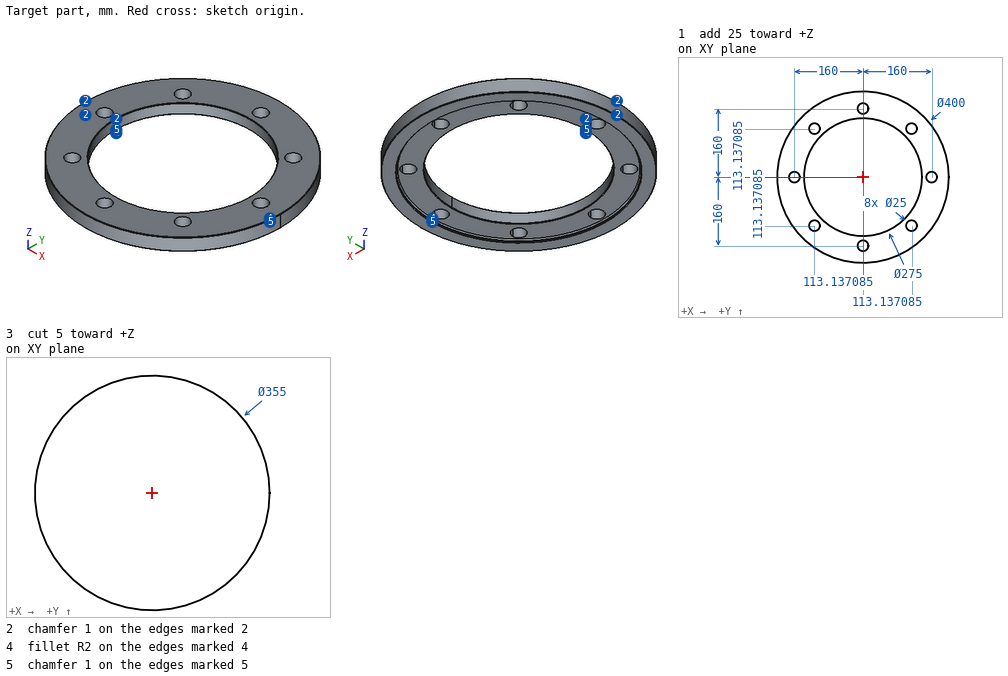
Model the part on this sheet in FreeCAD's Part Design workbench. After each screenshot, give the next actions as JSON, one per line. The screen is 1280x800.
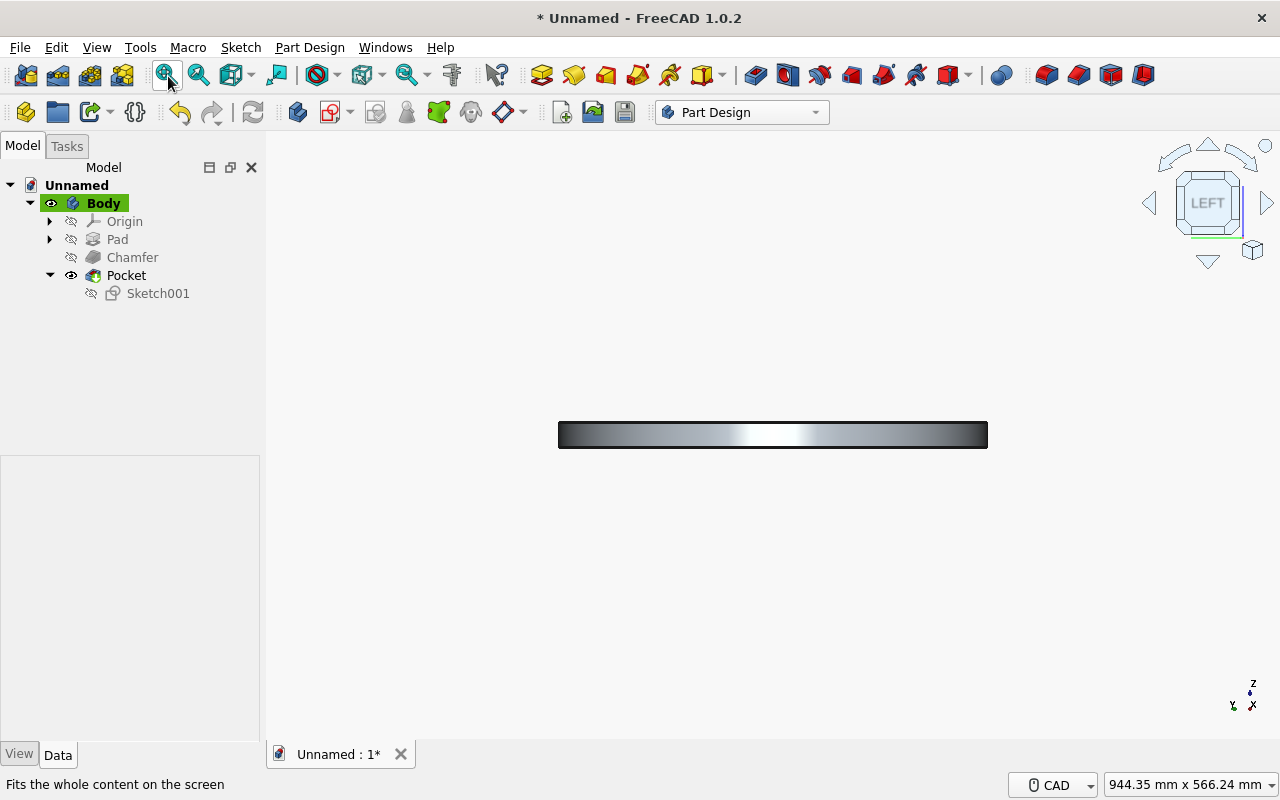
{"action": "left_click", "coordinate": [168, 76]}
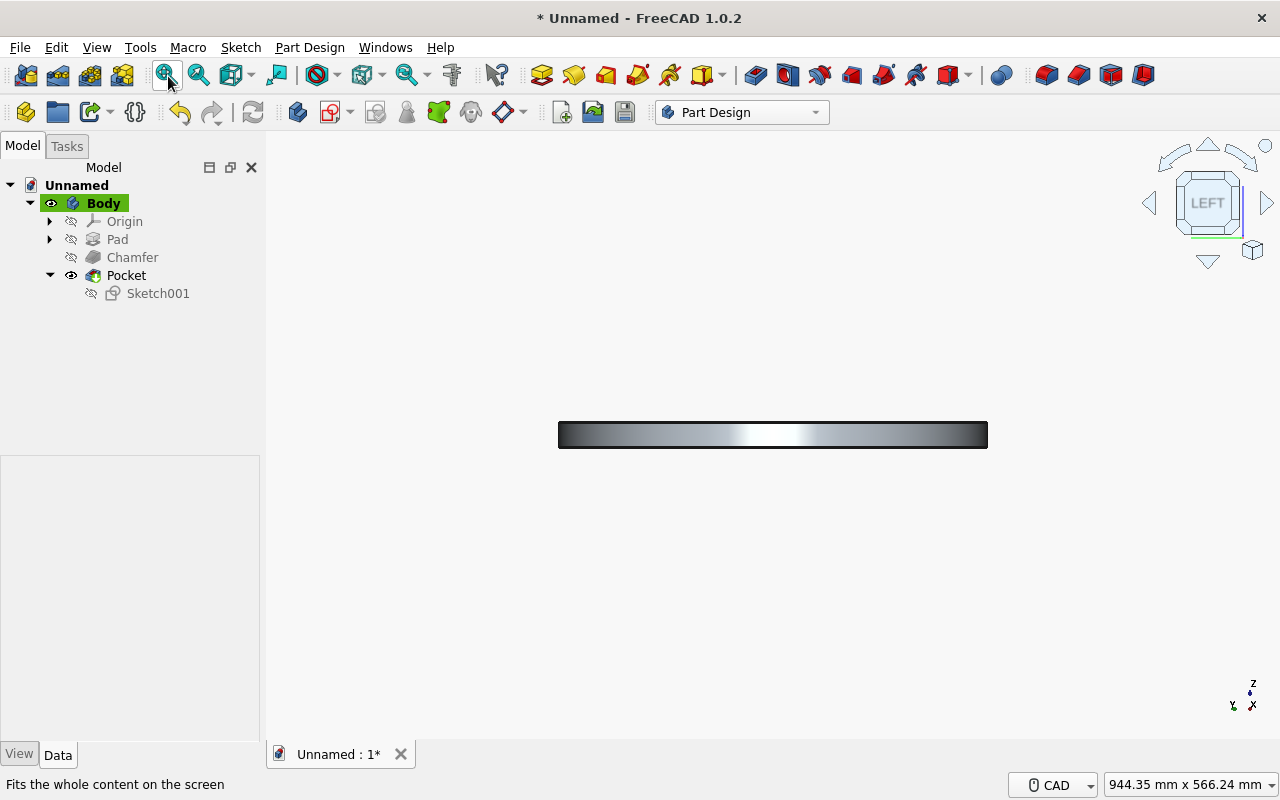
{"action": "key", "text": "v 3"}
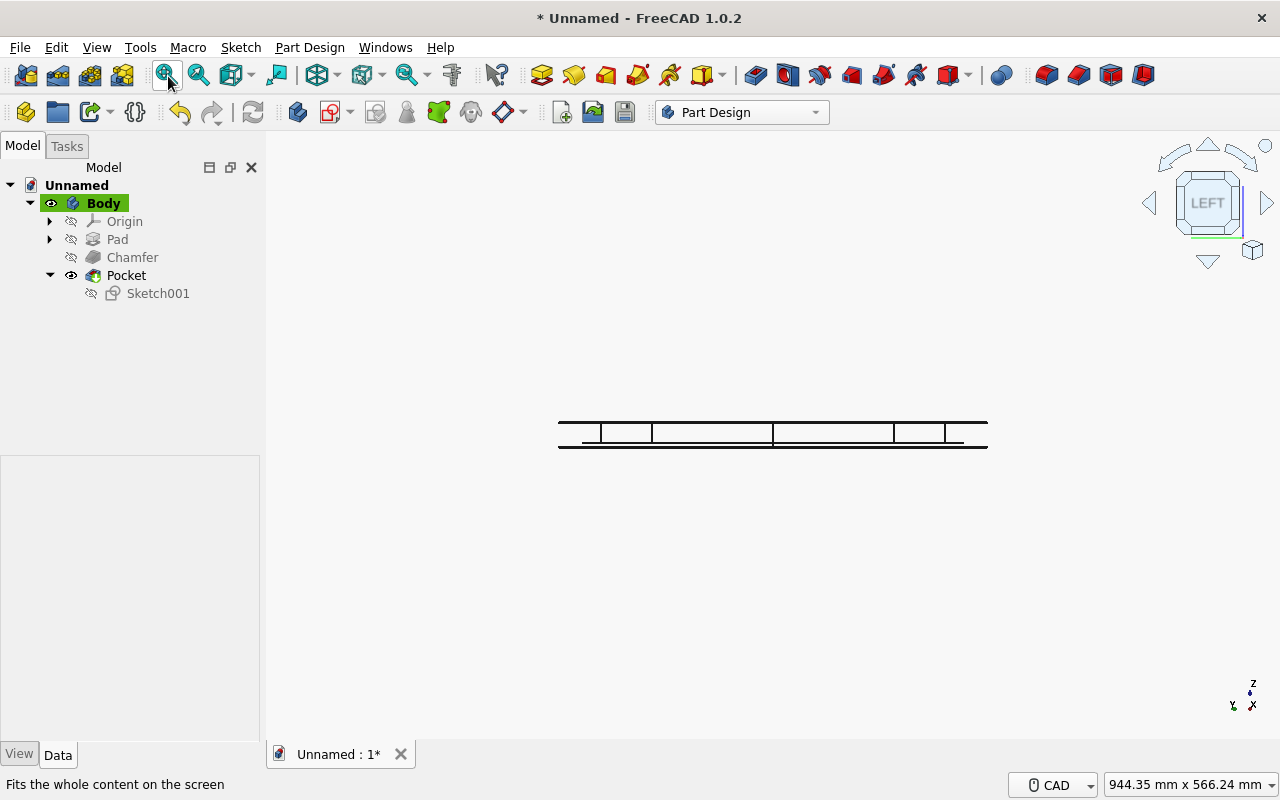
{"action": "key", "text": "0"}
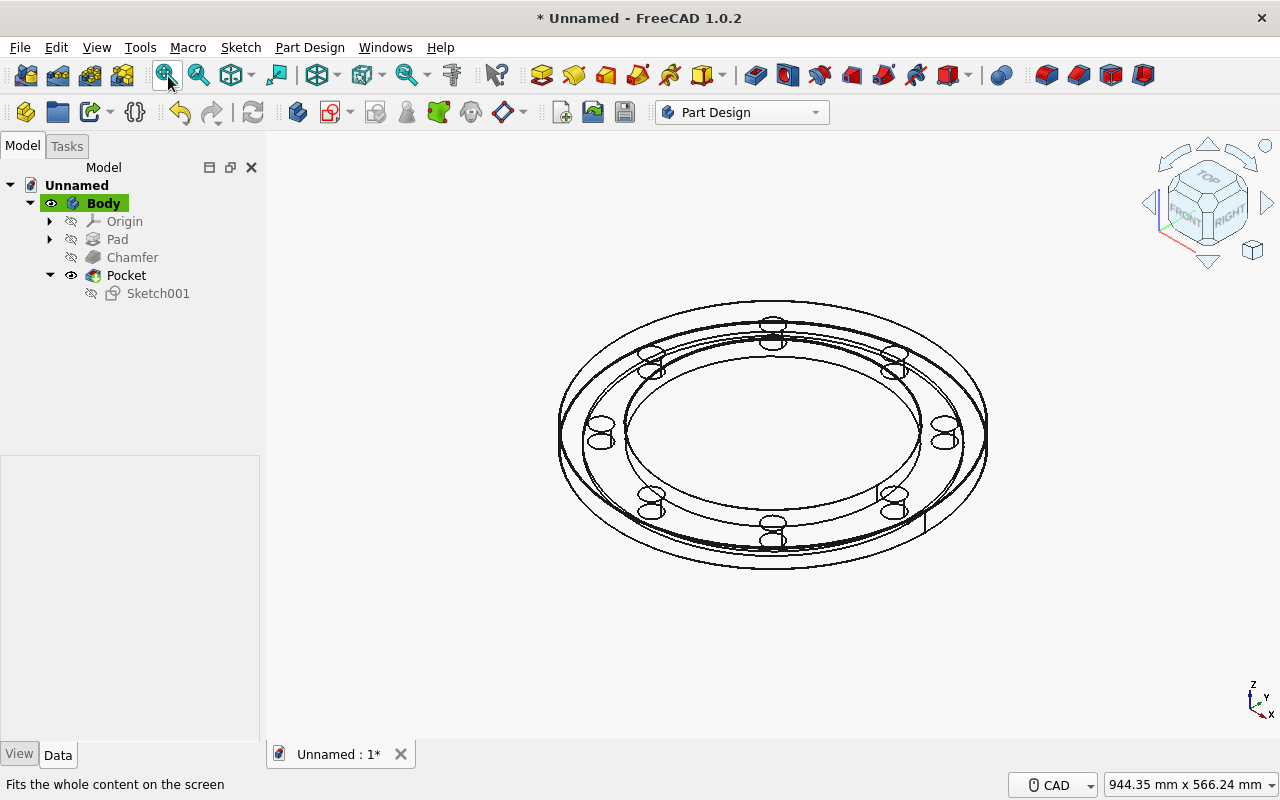
{"action": "left_click", "coordinate": [743, 332]}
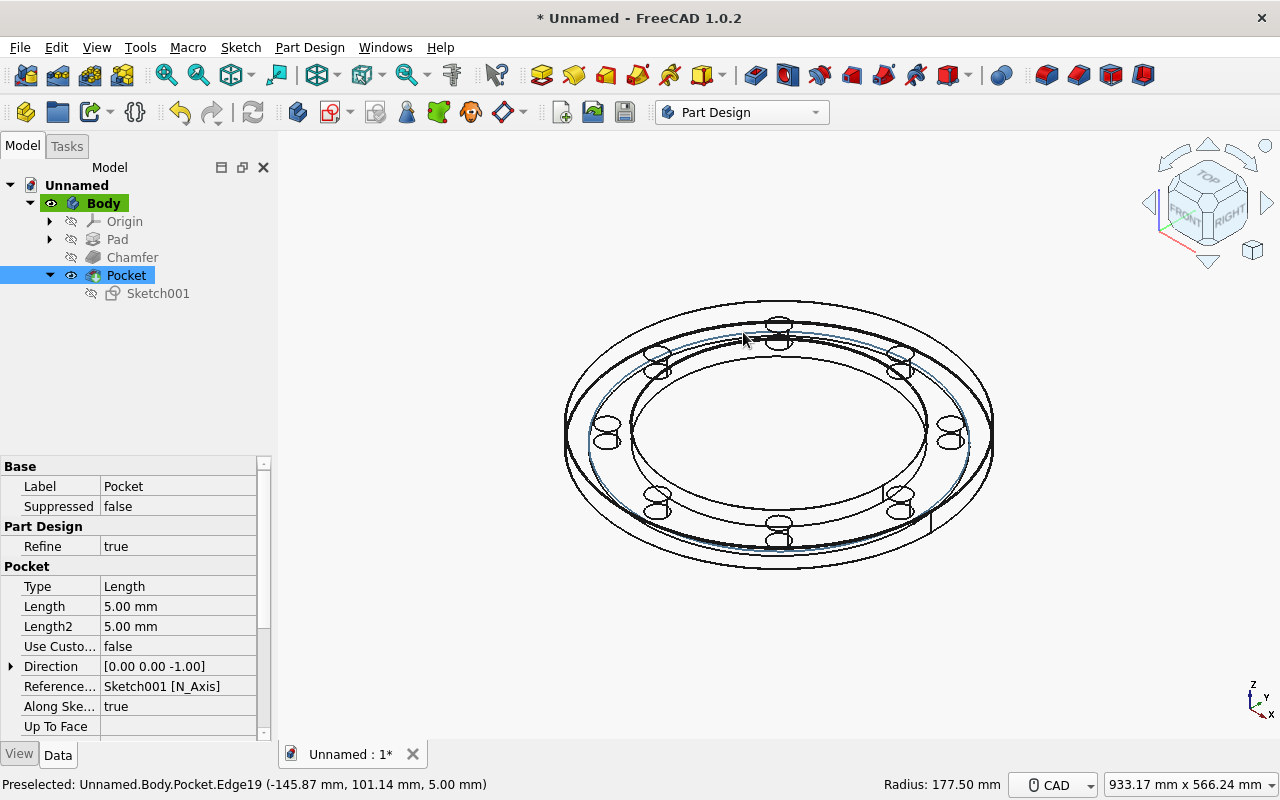
{"action": "key", "text": "v 1"}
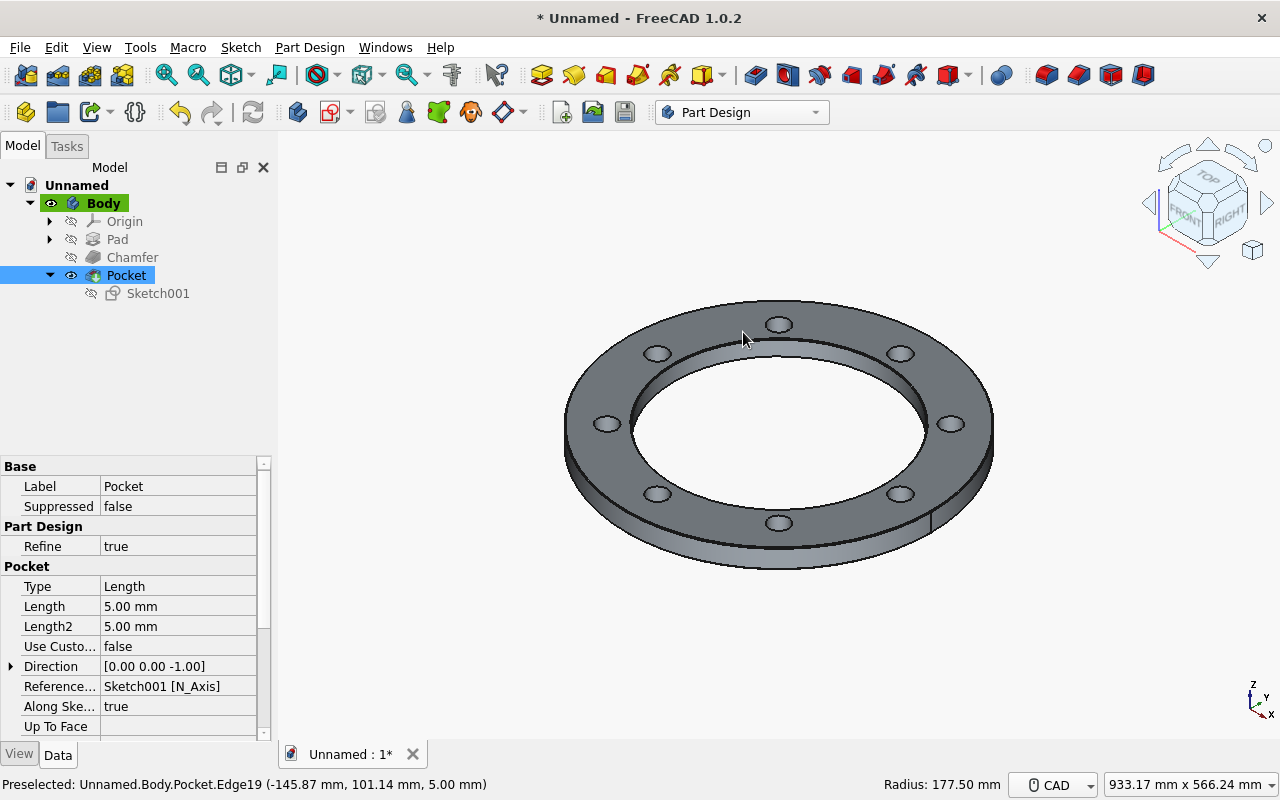
{"action": "left_click", "coordinate": [1048, 76]}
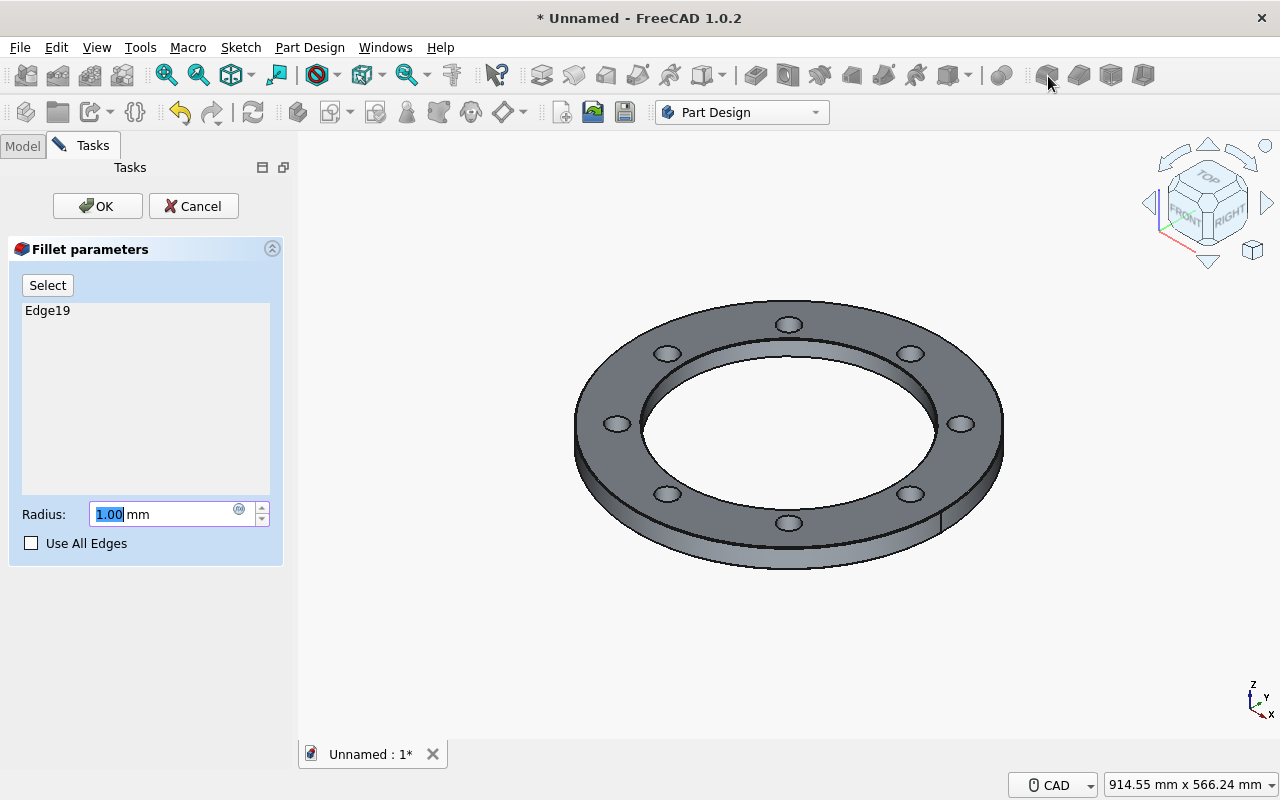
{"action": "type", "text": "2"}
{"action": "key", "text": "Tab"}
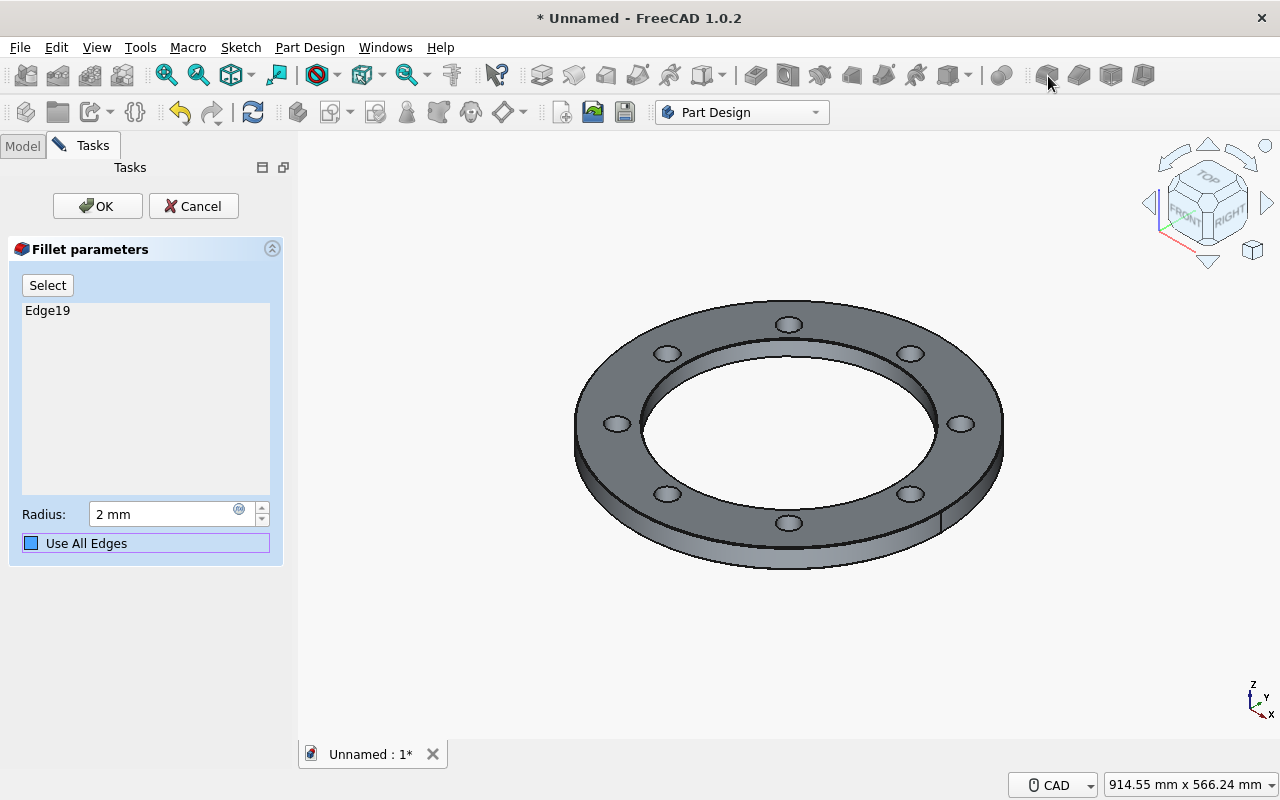
{"action": "left_click", "coordinate": [98, 206]}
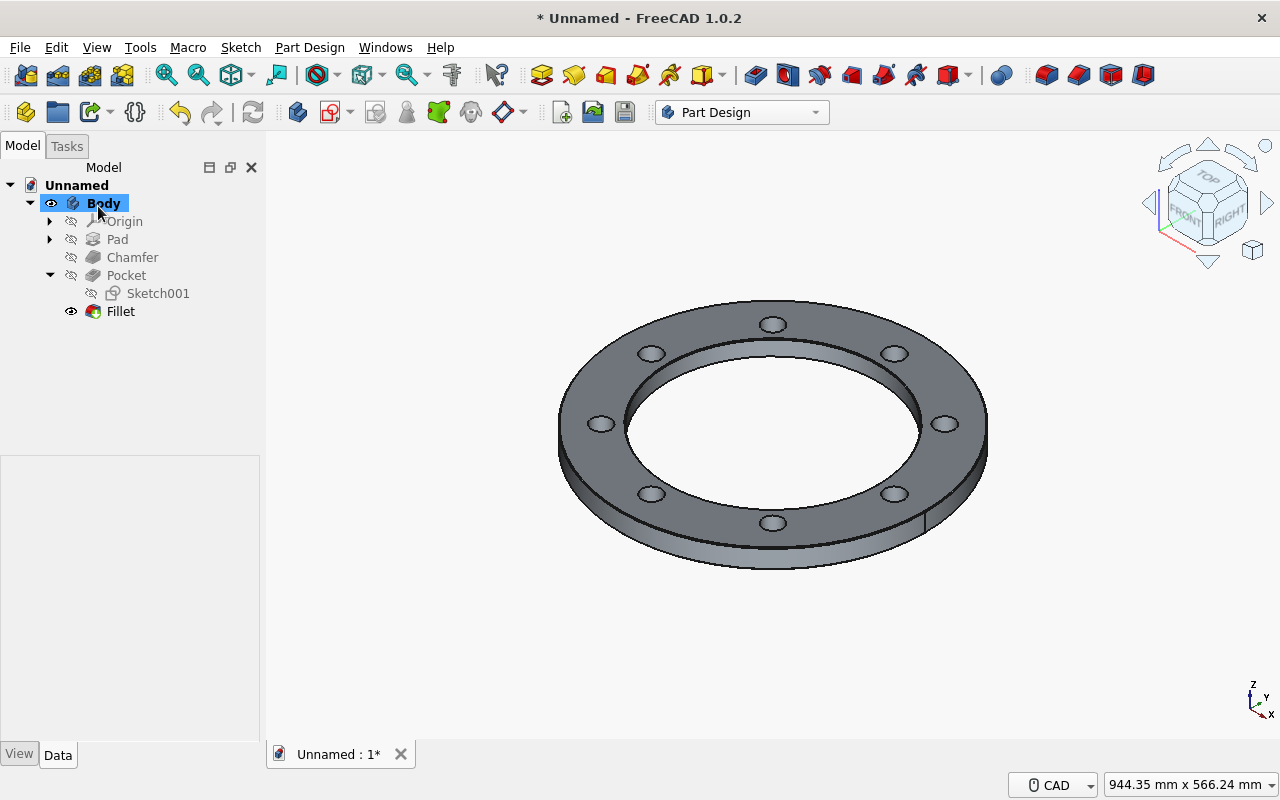
{"action": "key", "text": "2"}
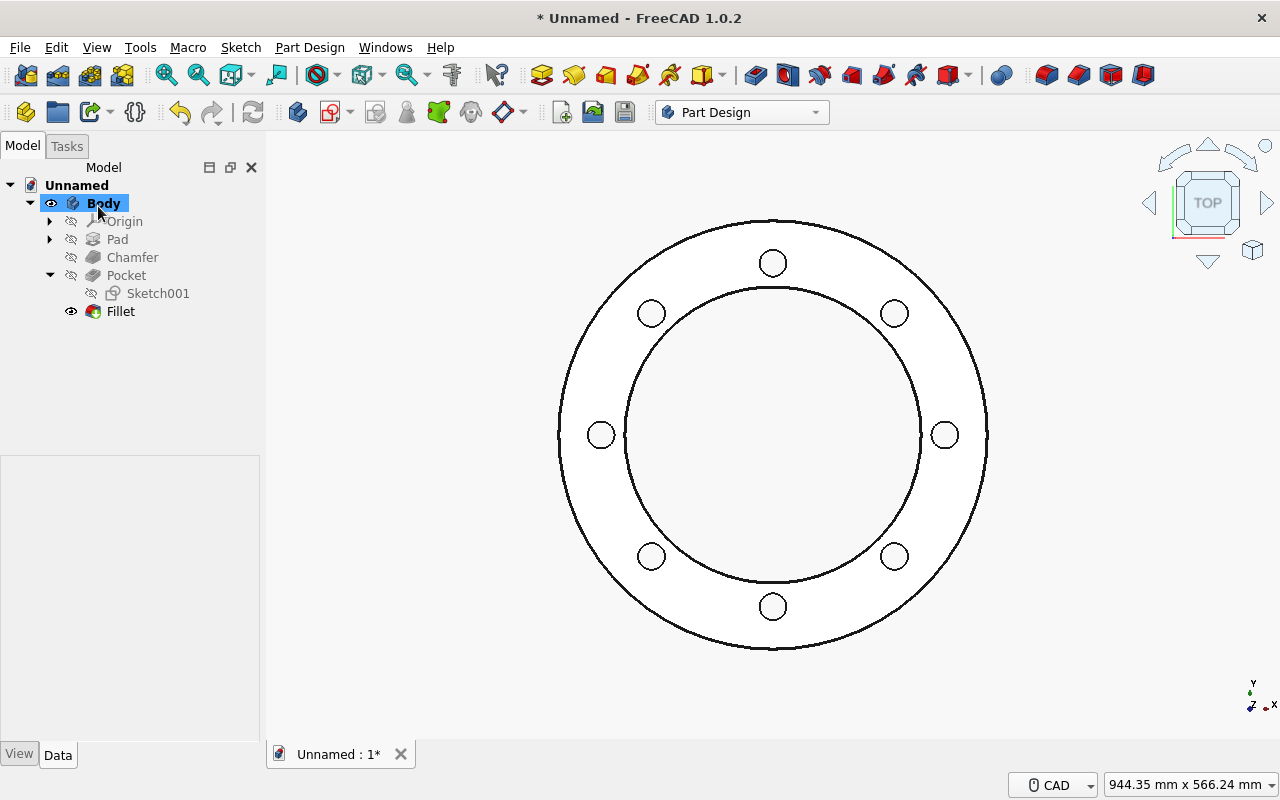
{"action": "key", "text": "0"}